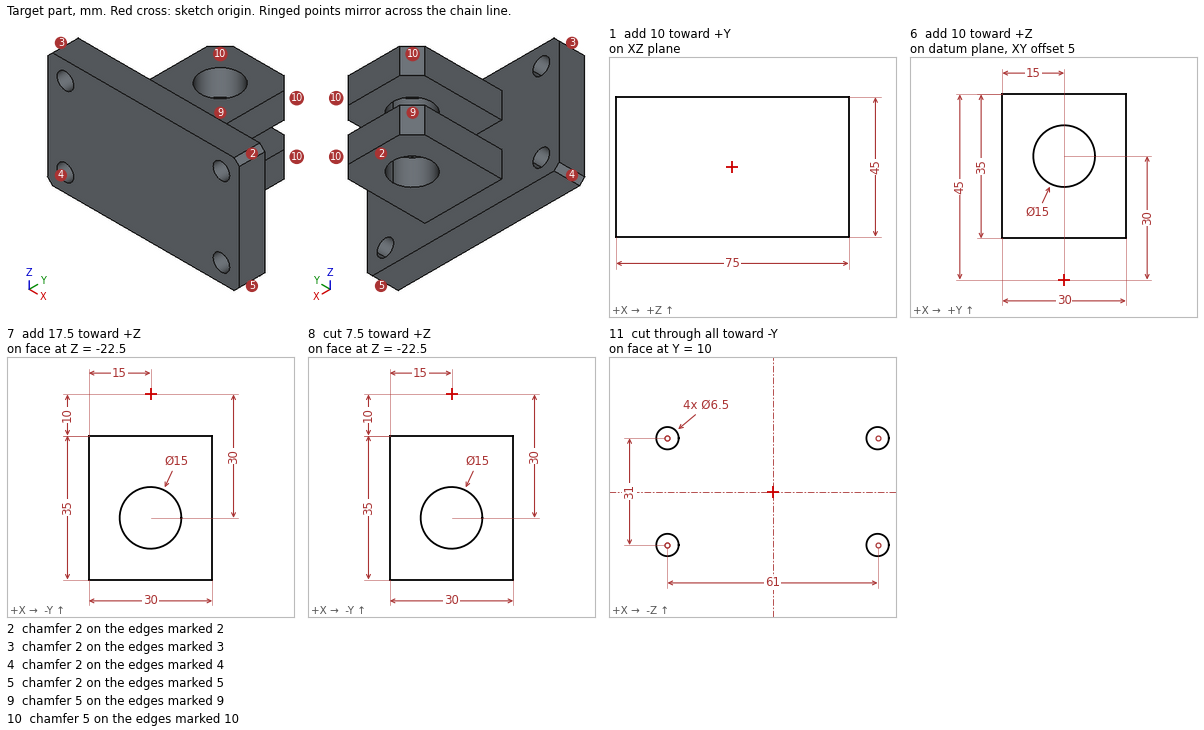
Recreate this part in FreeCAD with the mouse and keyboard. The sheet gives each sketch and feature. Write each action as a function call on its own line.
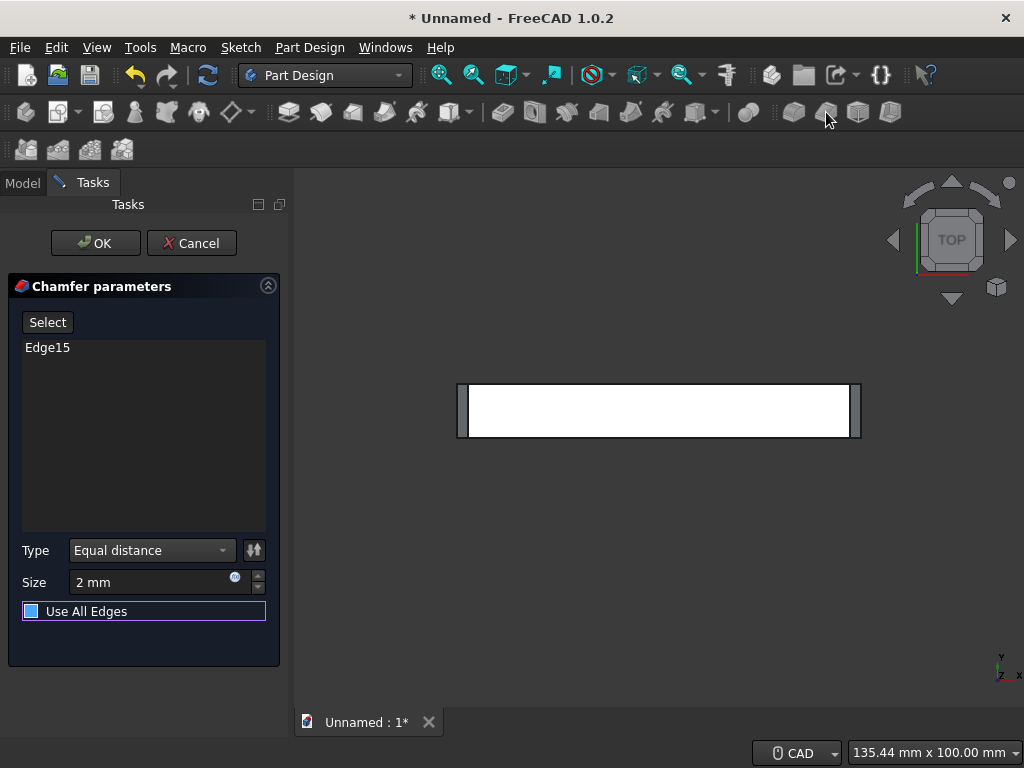
click(96, 243)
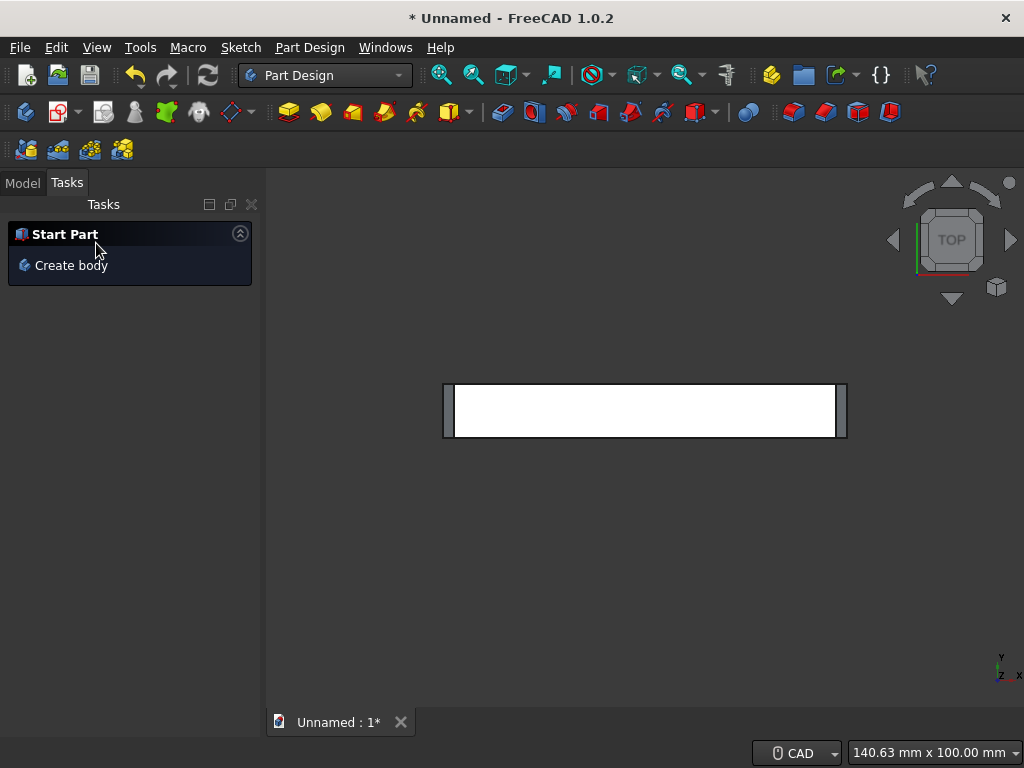
key(0)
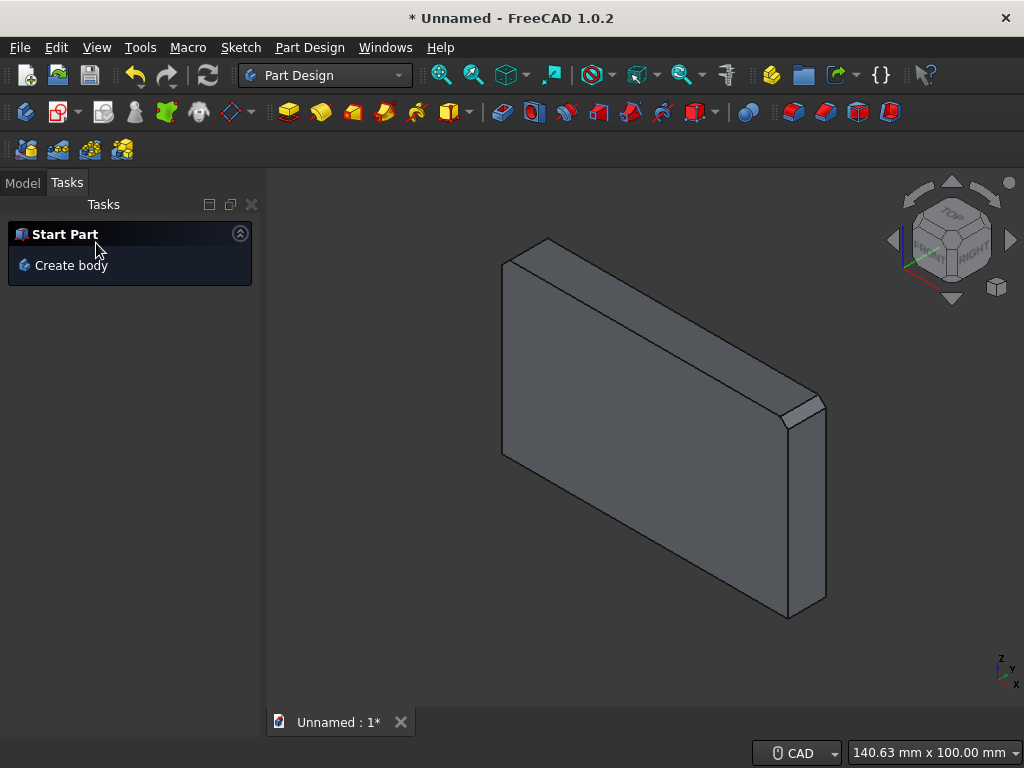
key(2)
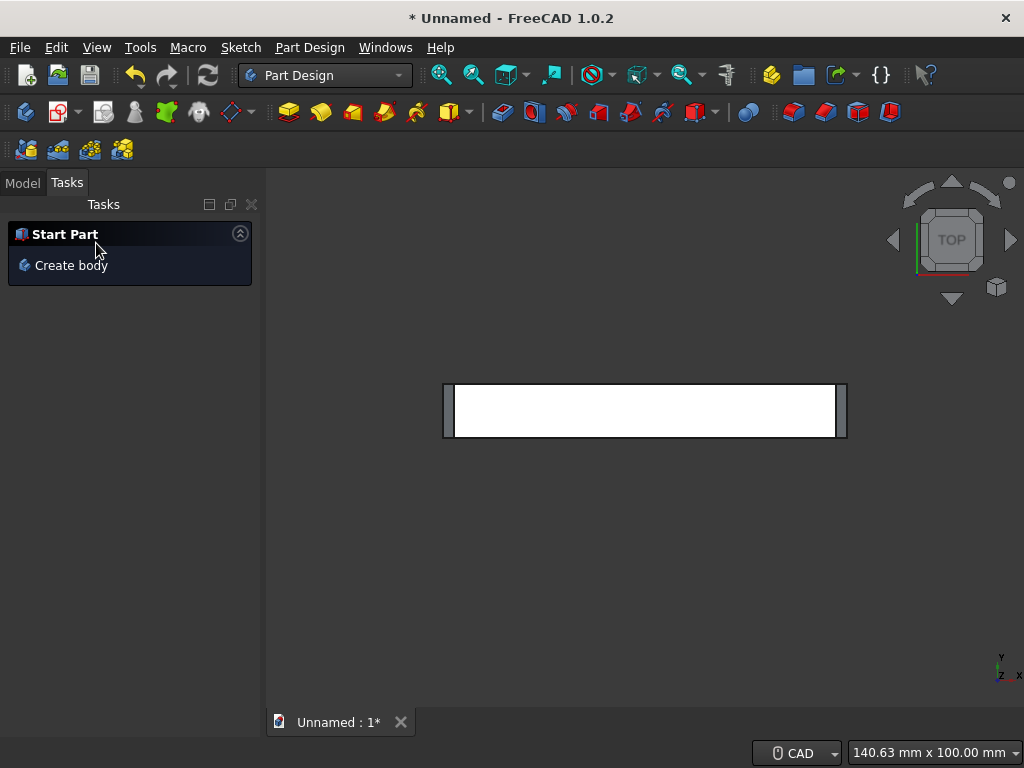
key(1)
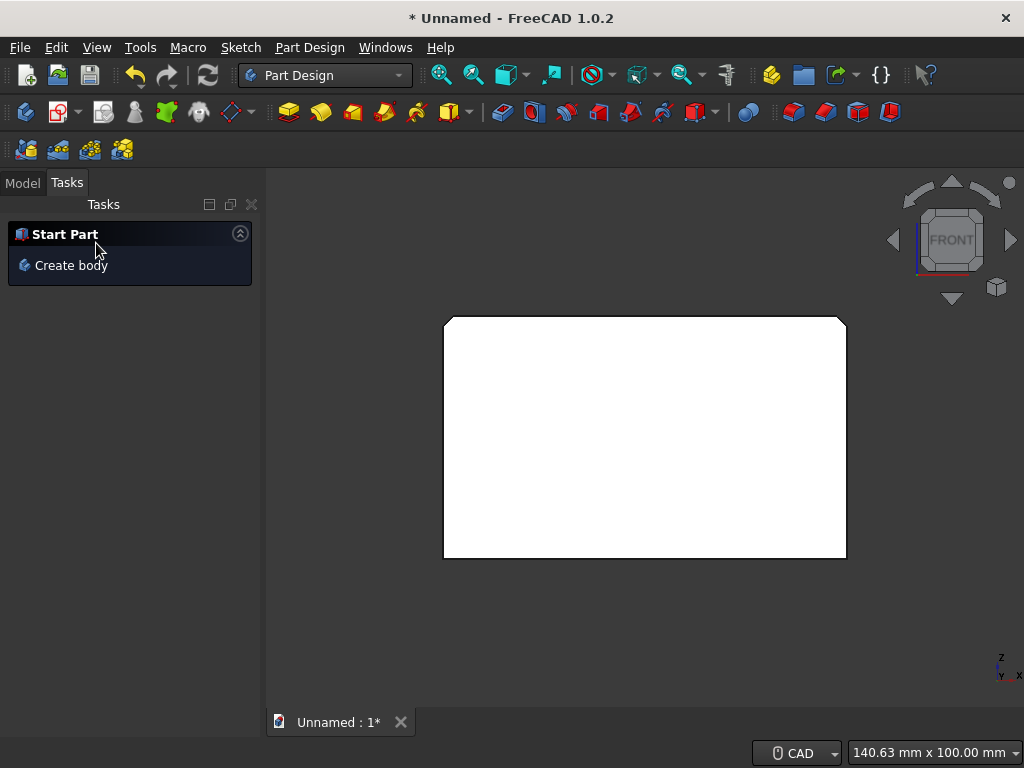
key(3)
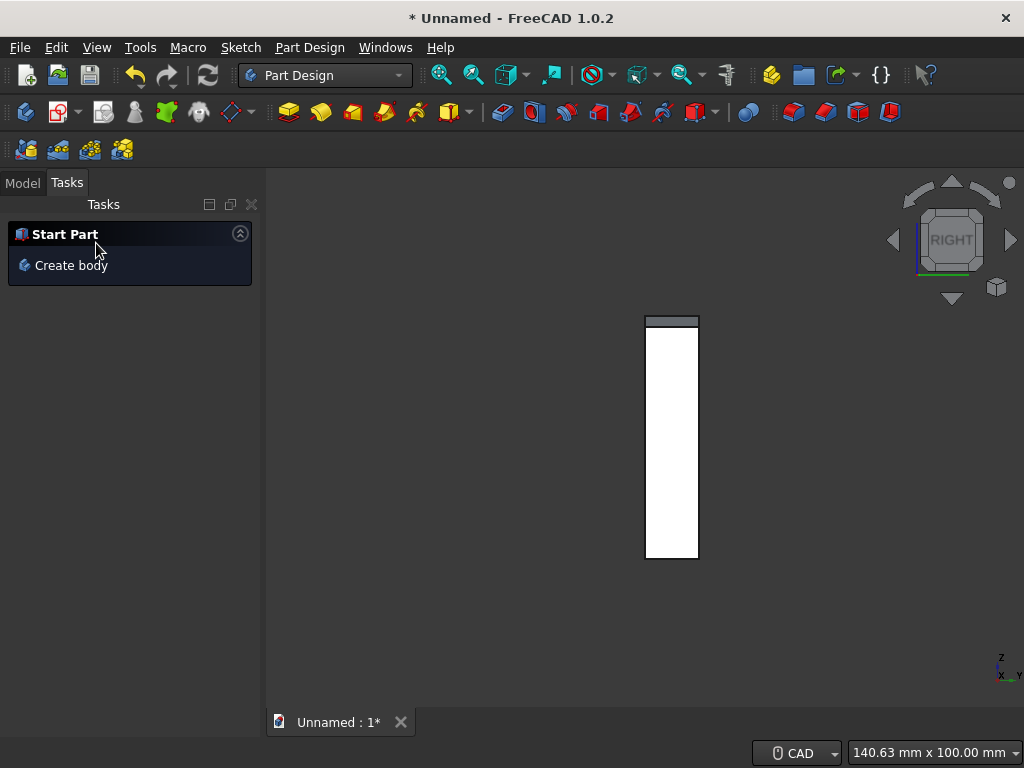
key(5)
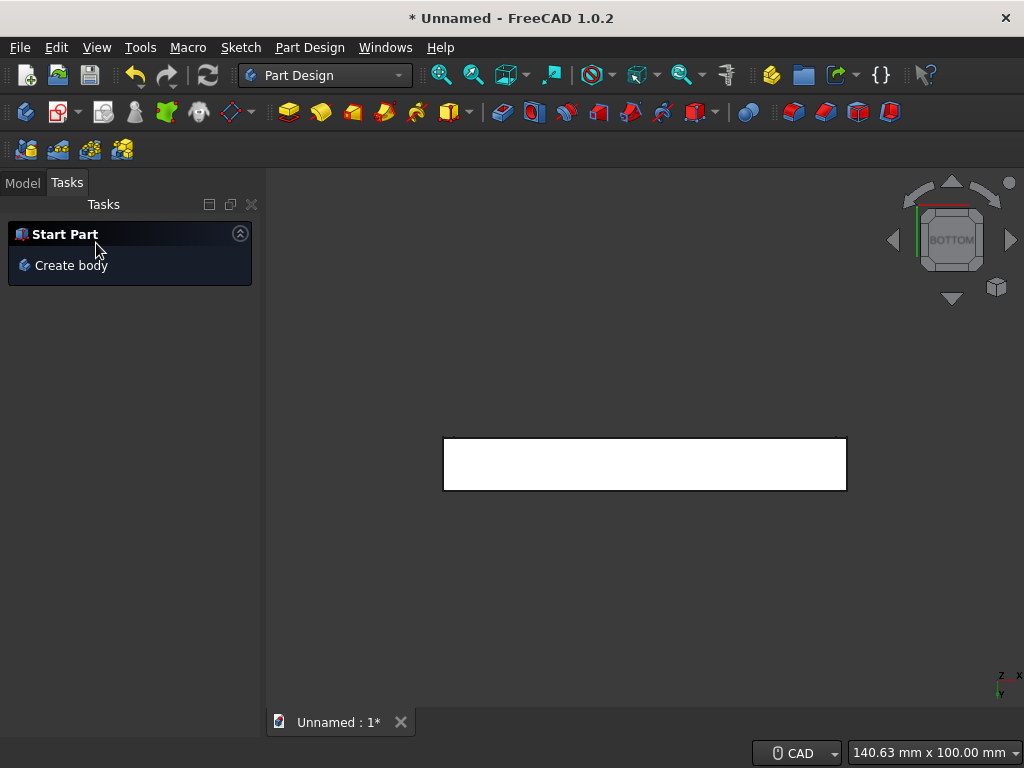
click(443, 463)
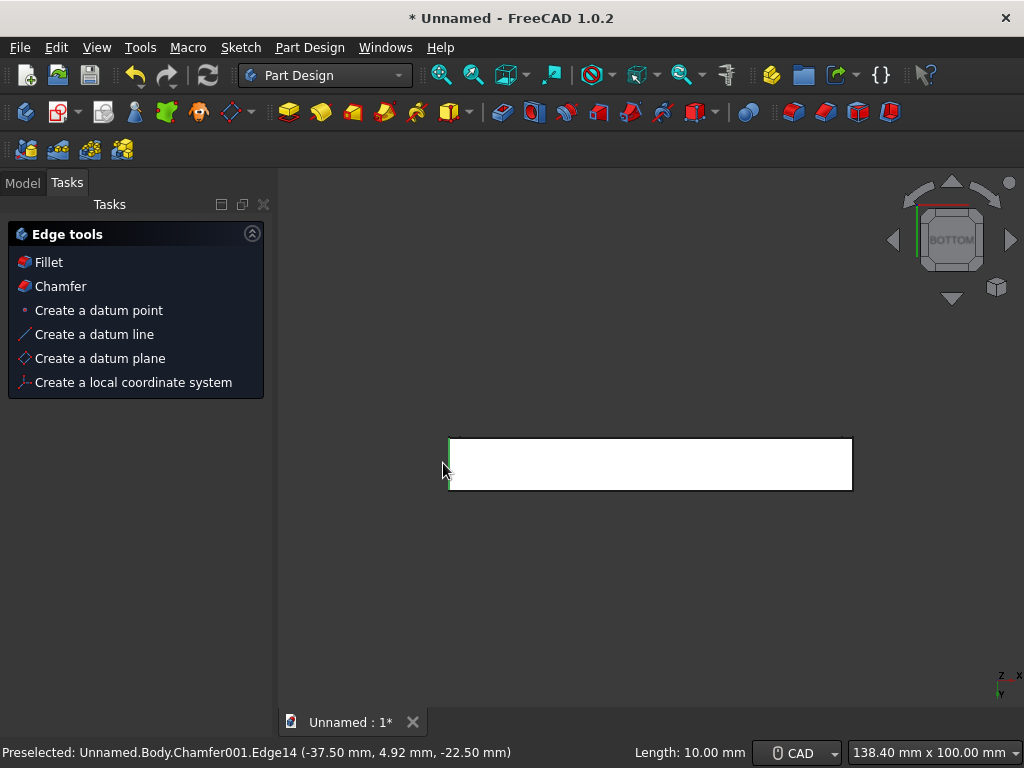
click(826, 112)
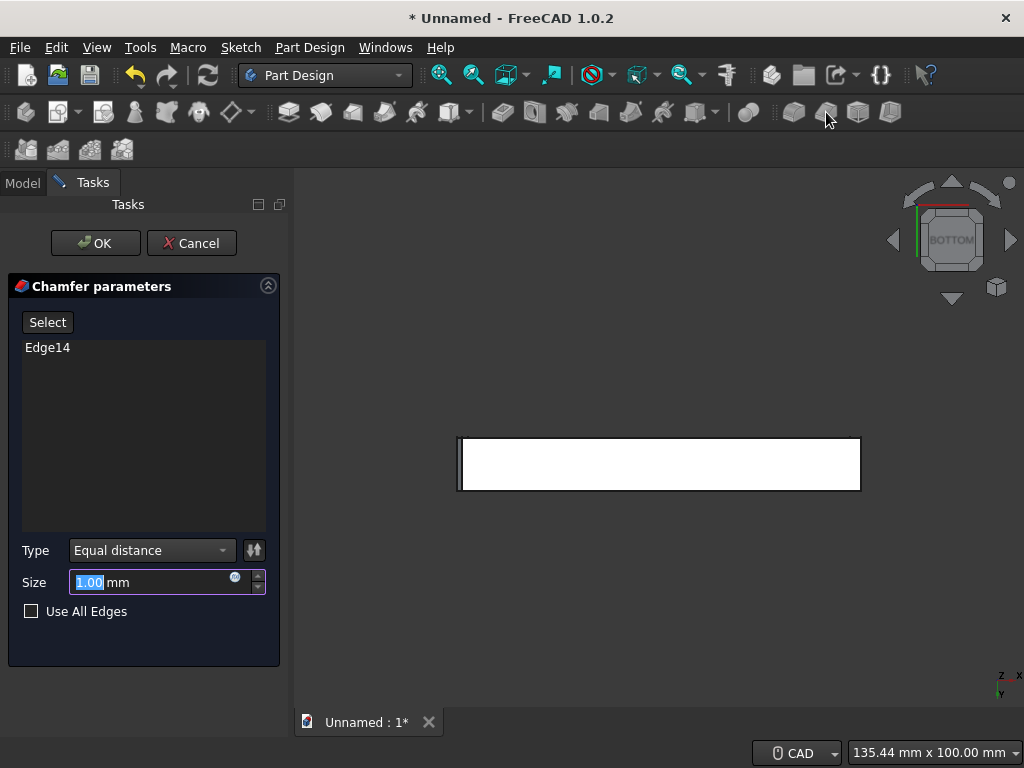
text(2)
key(Tab)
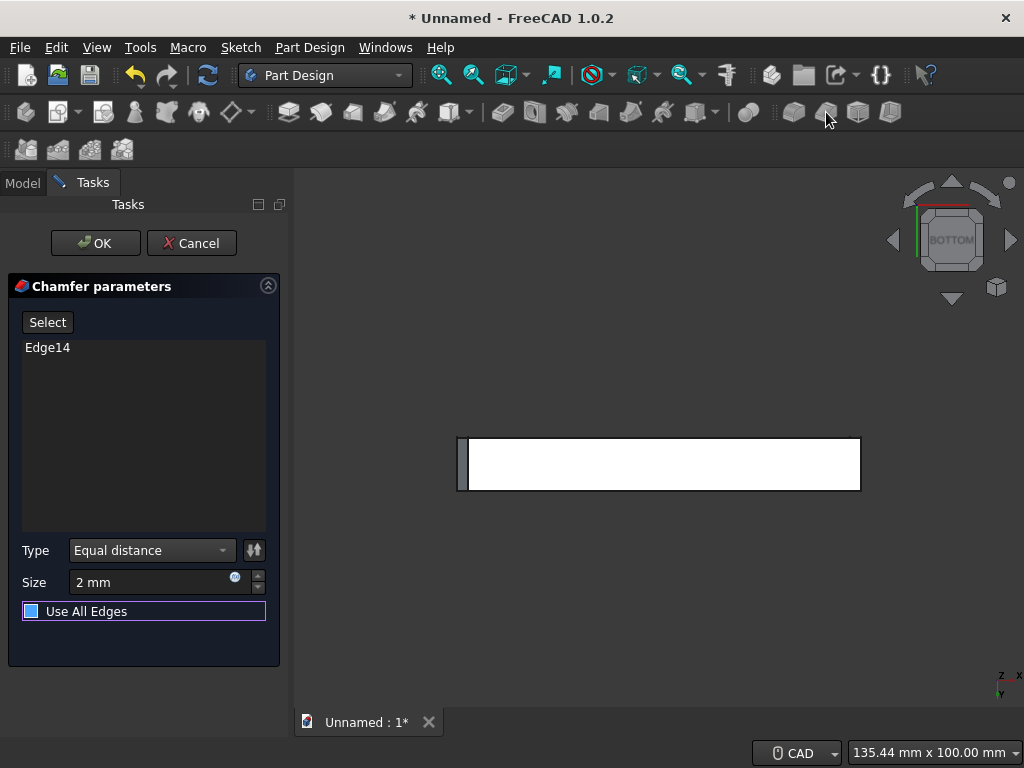
click(96, 243)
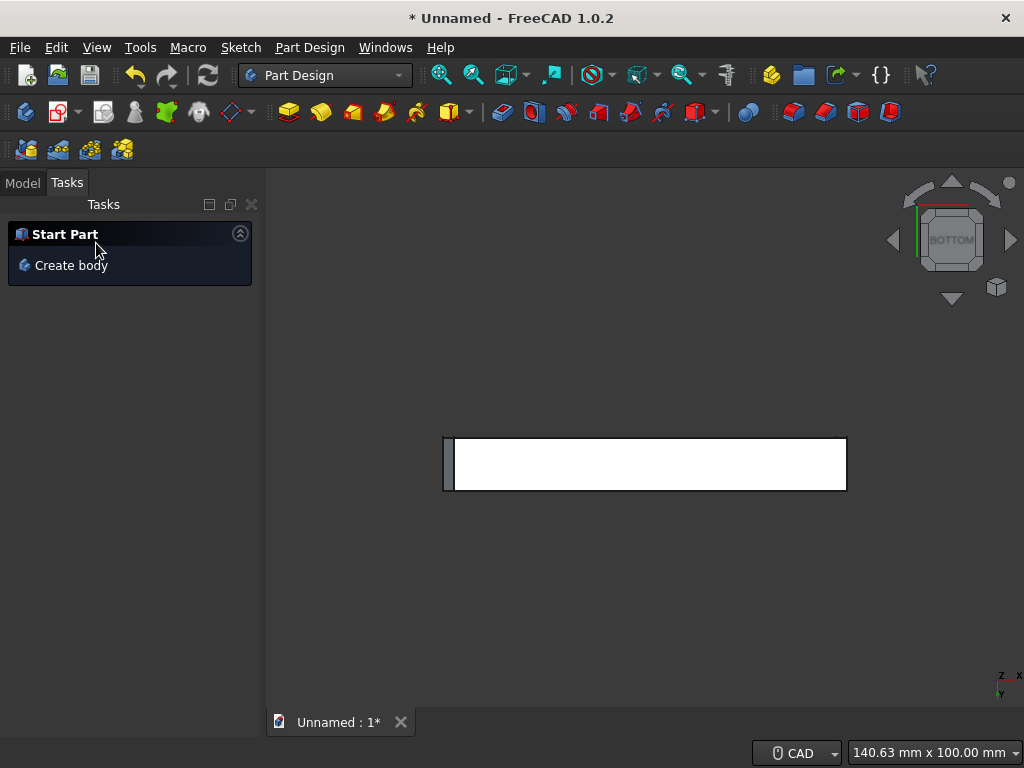
click(847, 463)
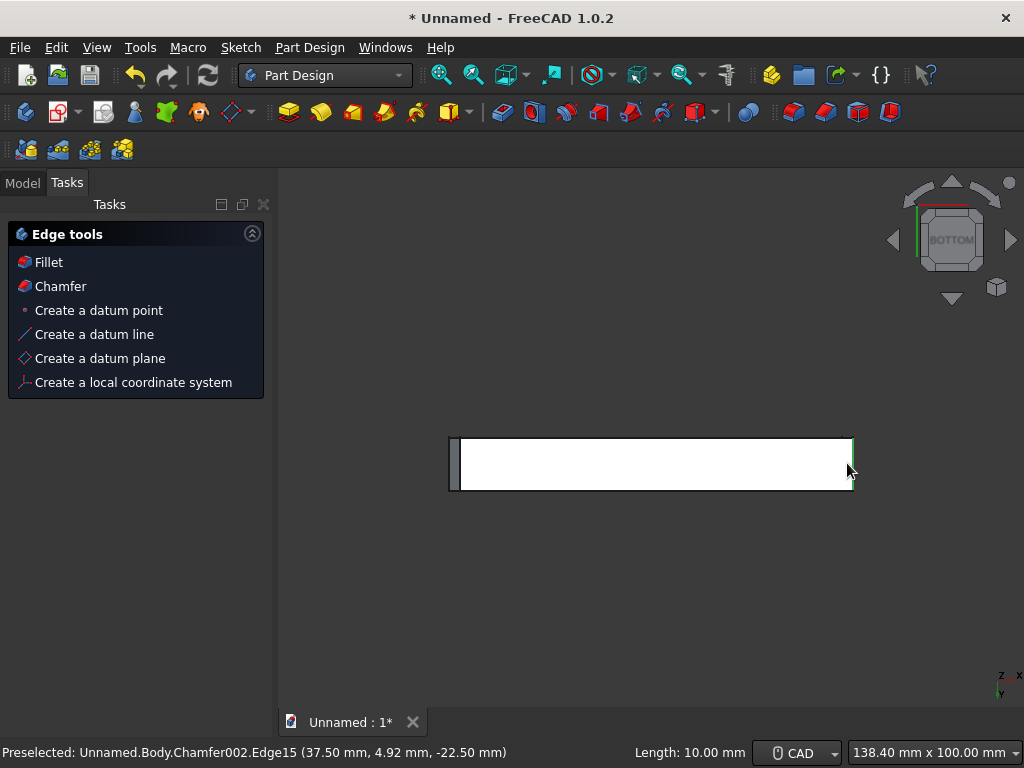
click(826, 112)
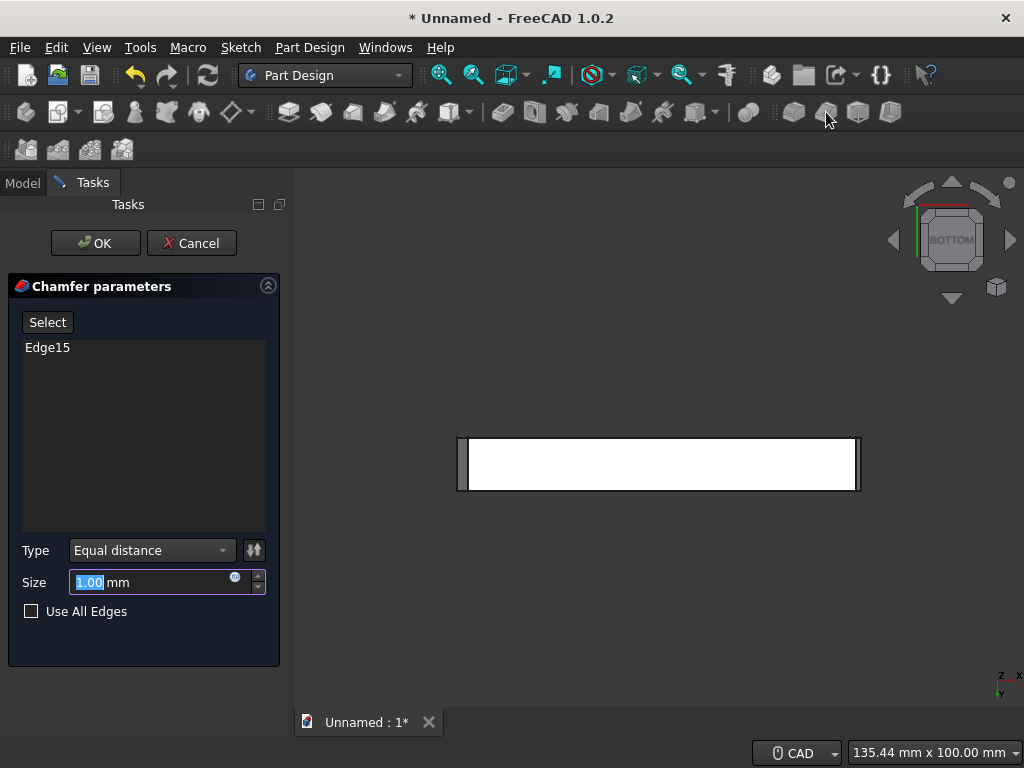
text(2)
key(Tab)